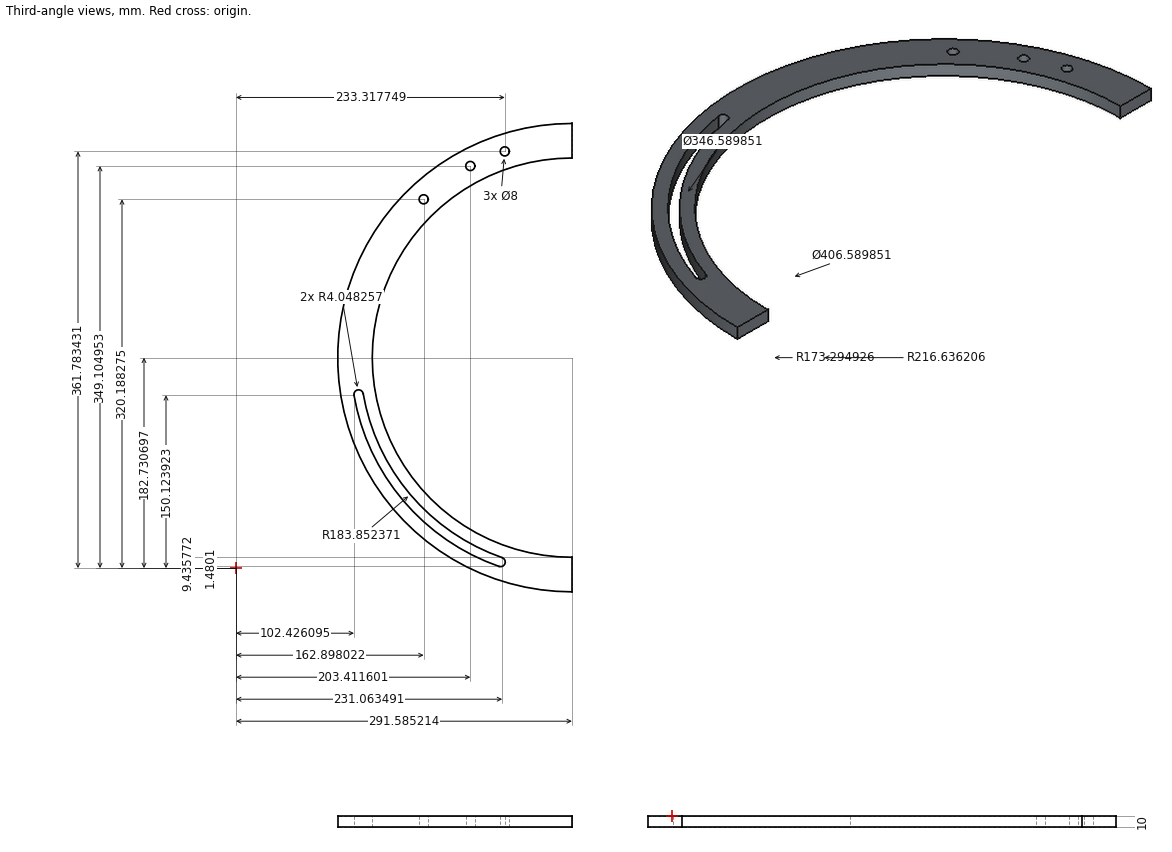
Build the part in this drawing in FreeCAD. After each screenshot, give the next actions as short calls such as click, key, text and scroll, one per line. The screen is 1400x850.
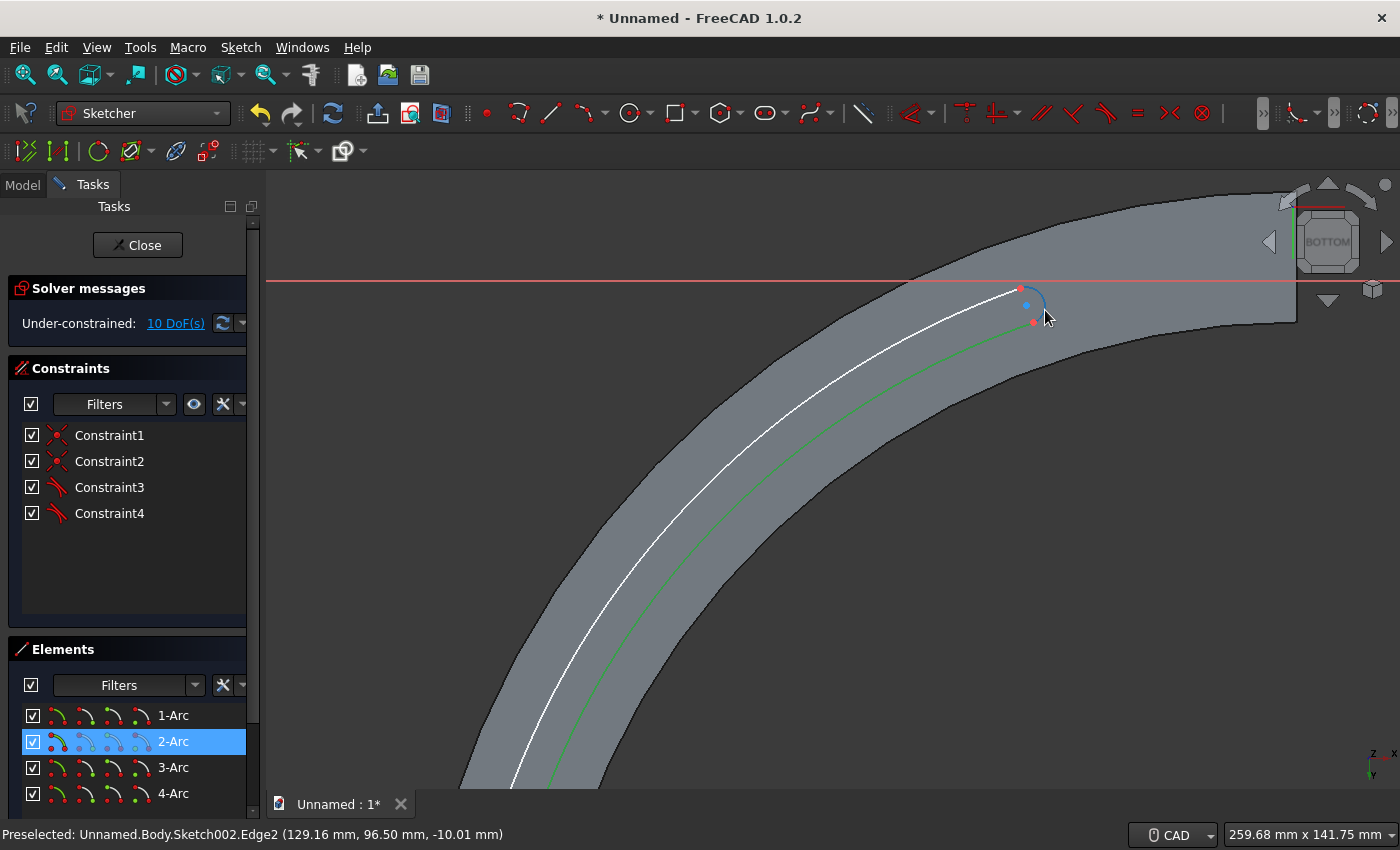
click(1044, 311)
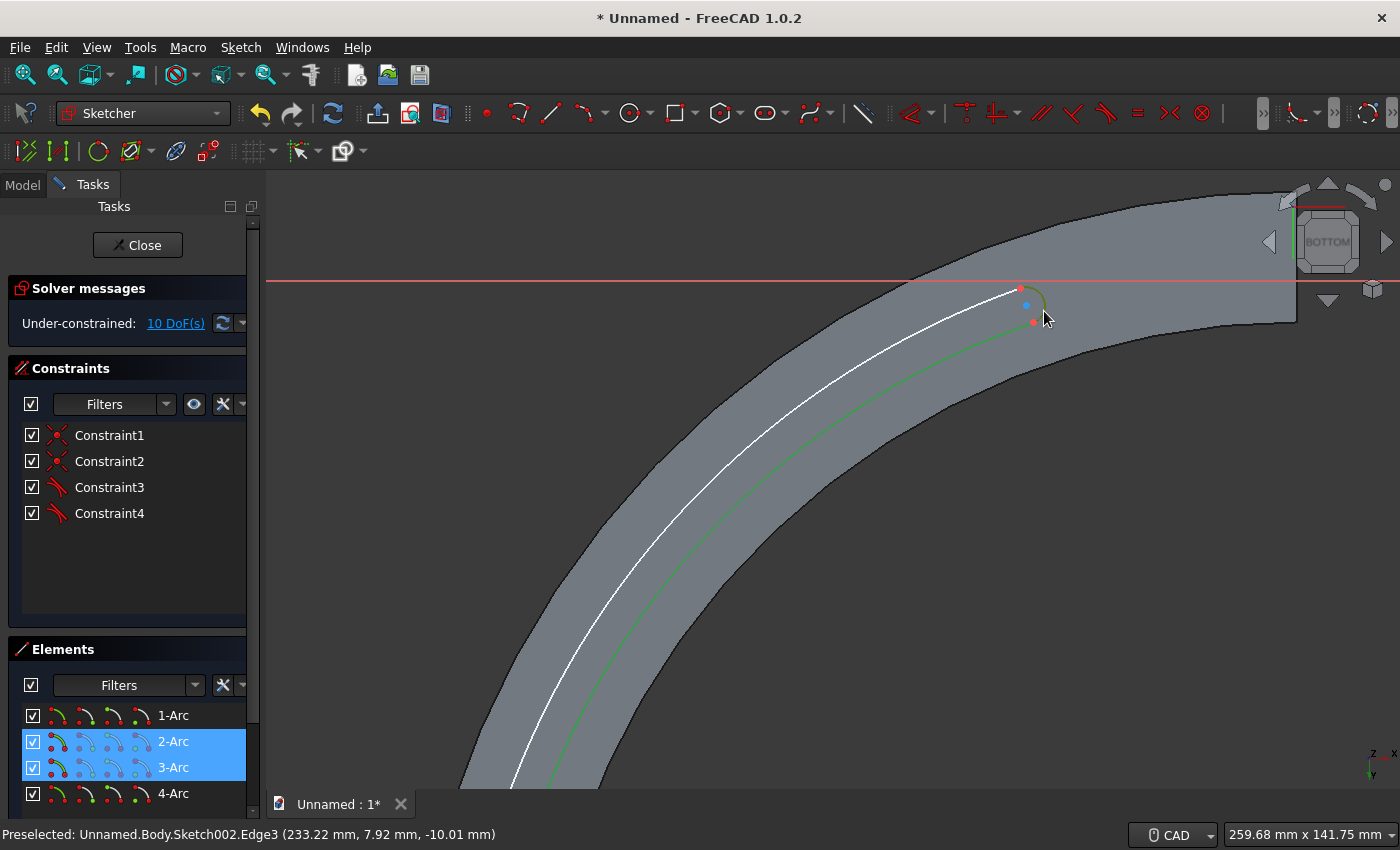
click(1106, 114)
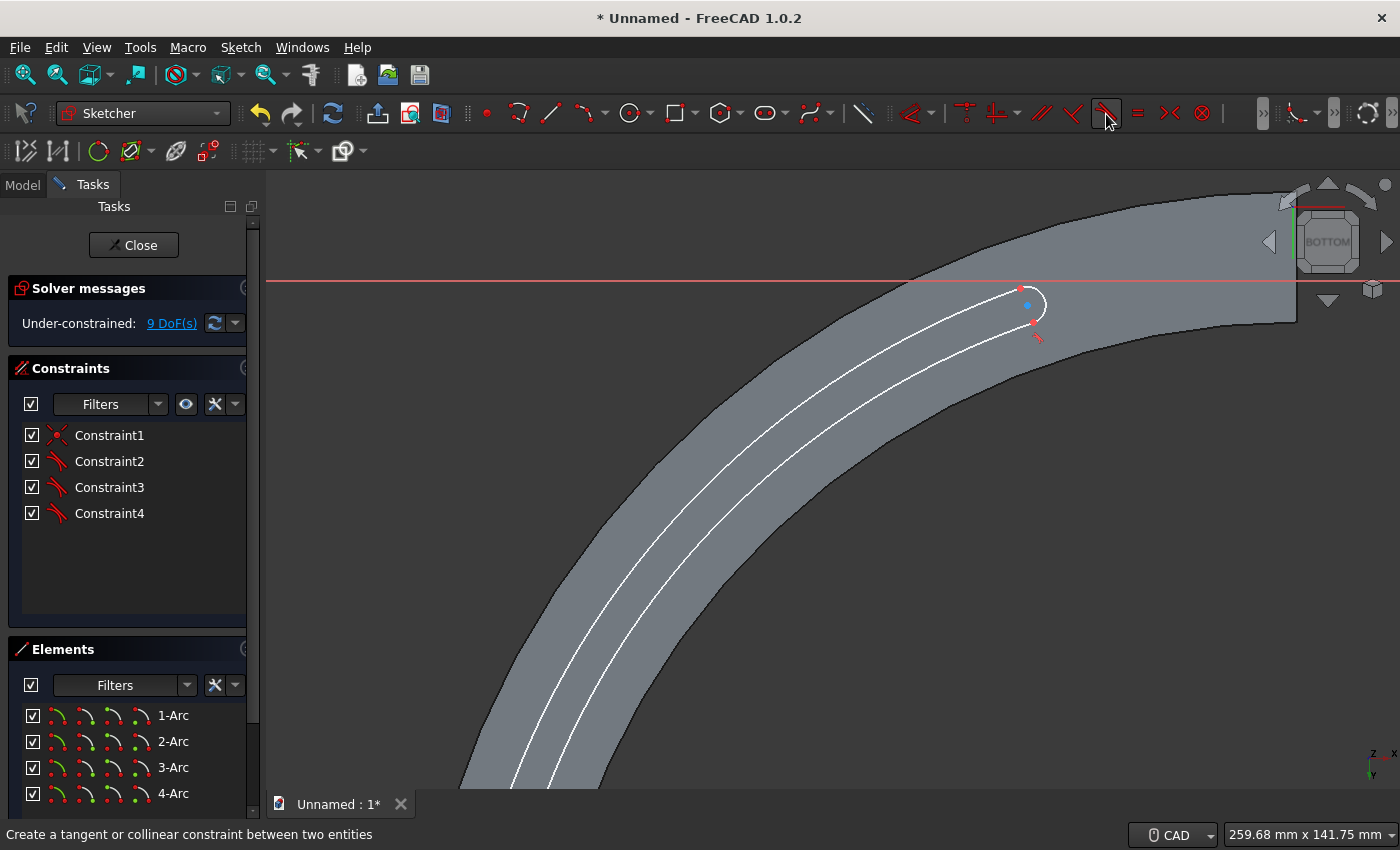
click(1045, 311)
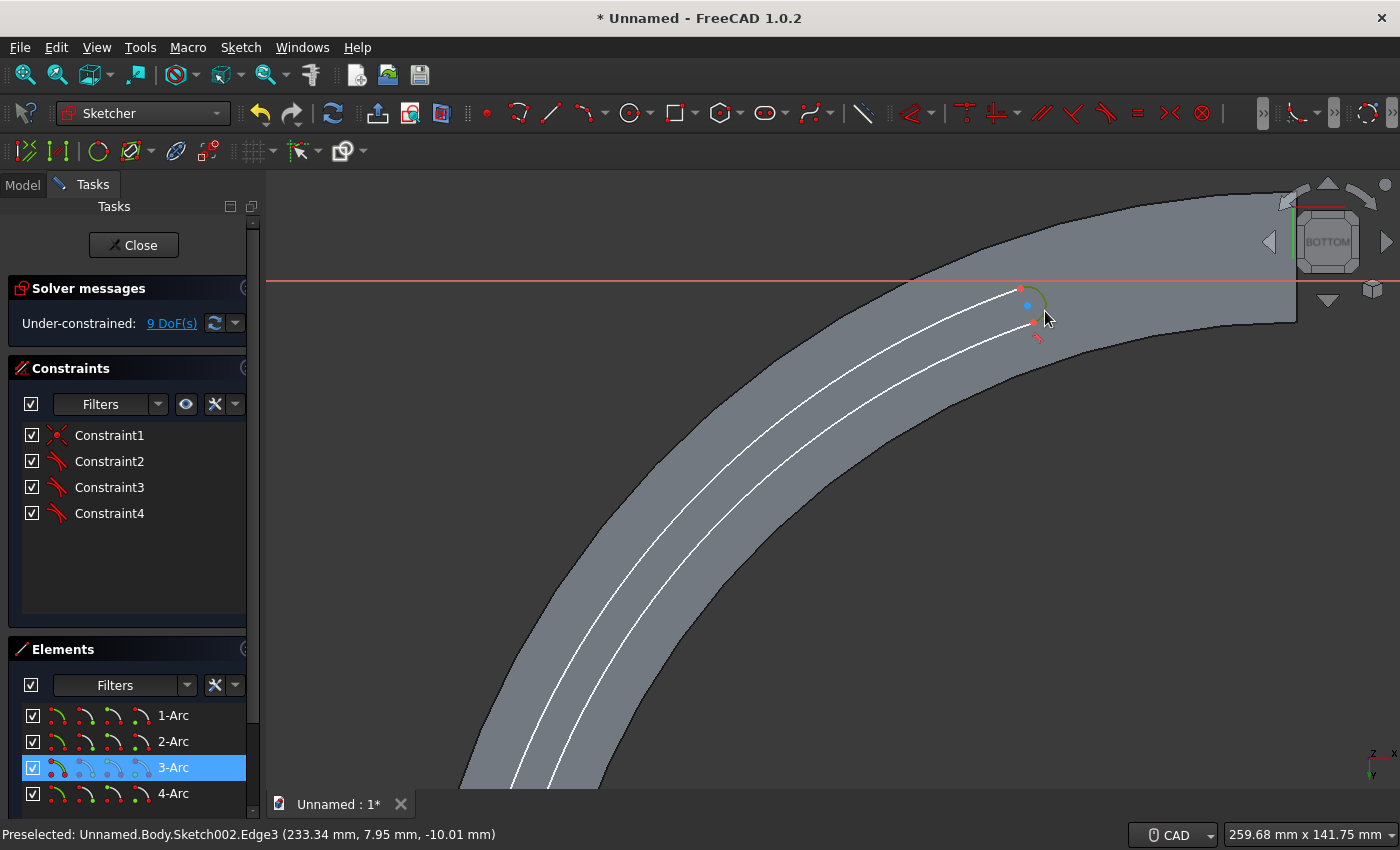
click(786, 416)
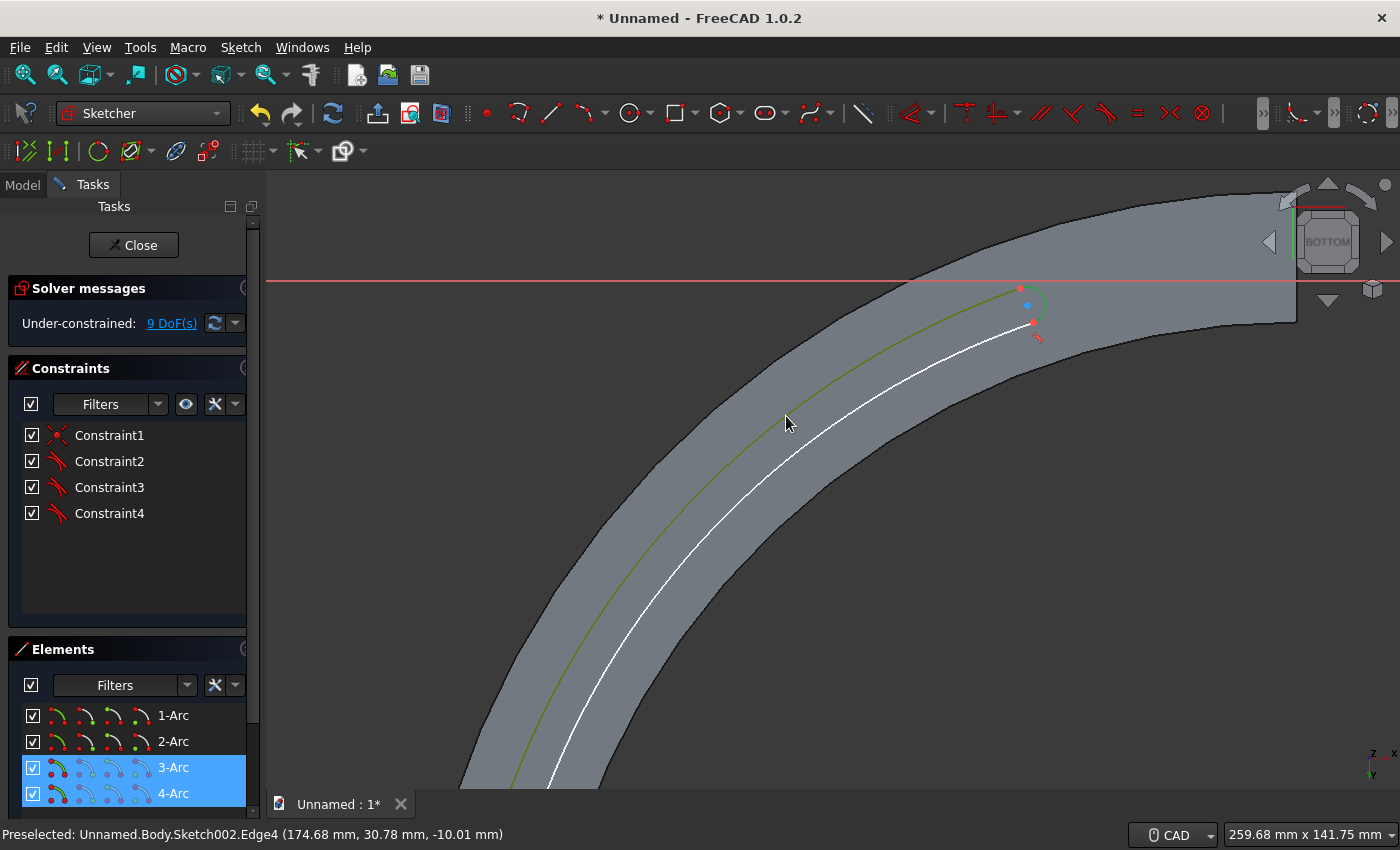
key(t)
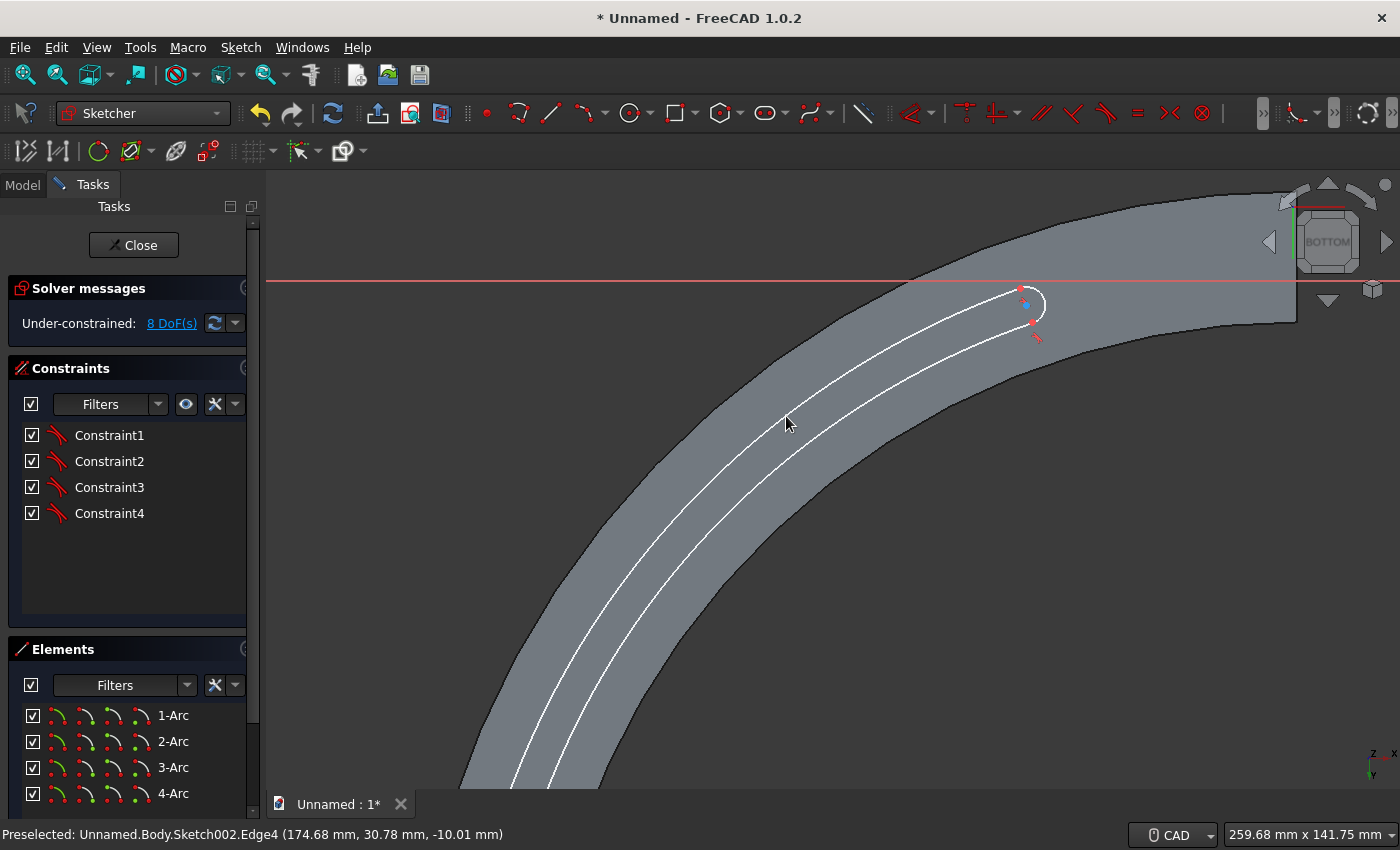
click(807, 444)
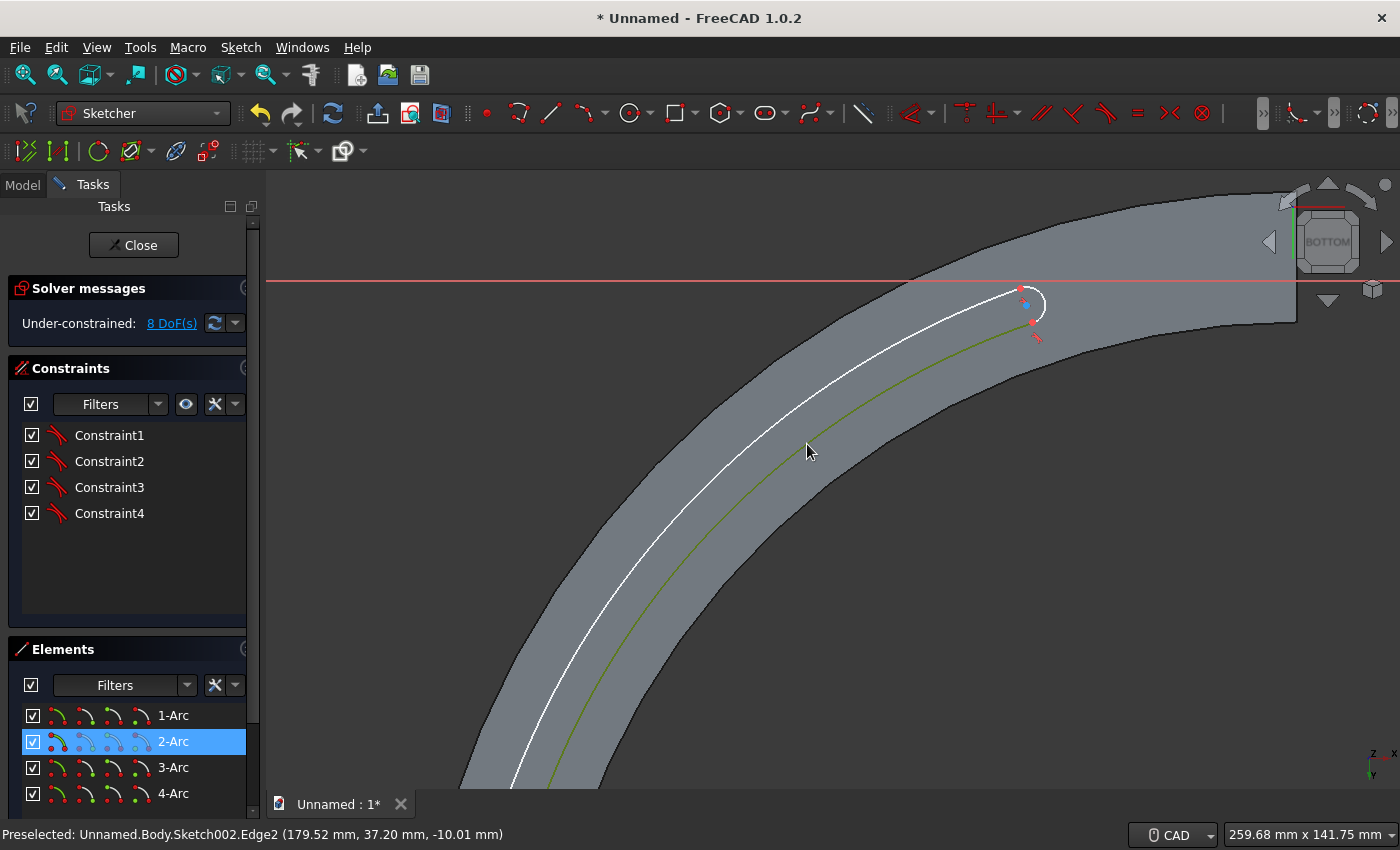
click(786, 416)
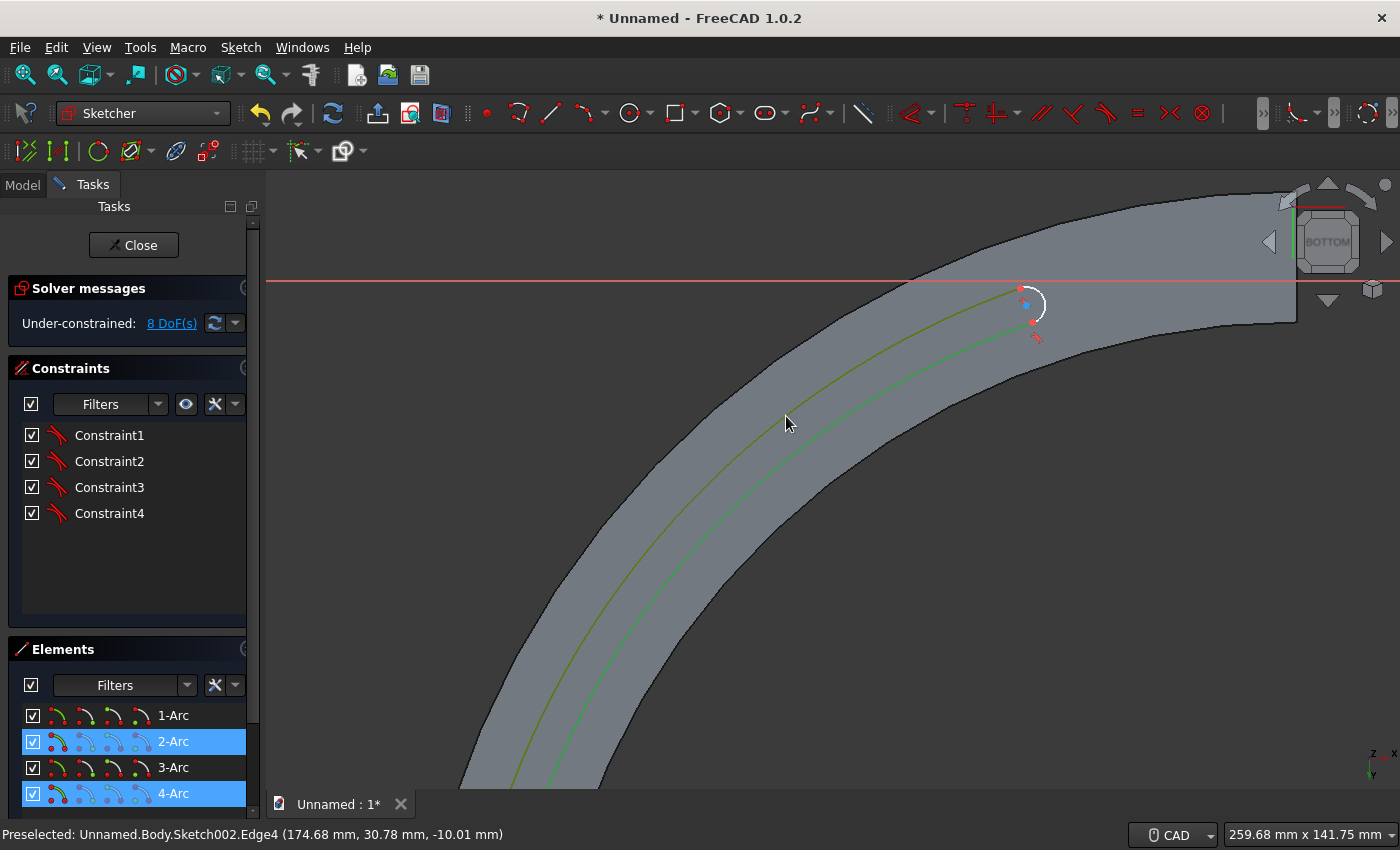
click(966, 114)